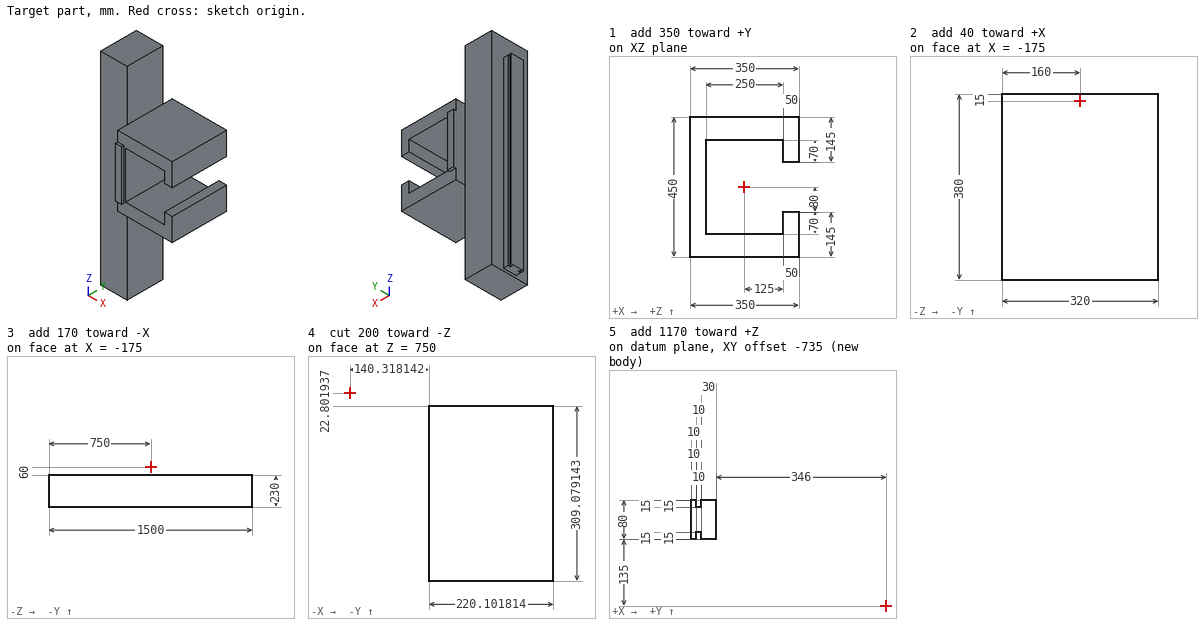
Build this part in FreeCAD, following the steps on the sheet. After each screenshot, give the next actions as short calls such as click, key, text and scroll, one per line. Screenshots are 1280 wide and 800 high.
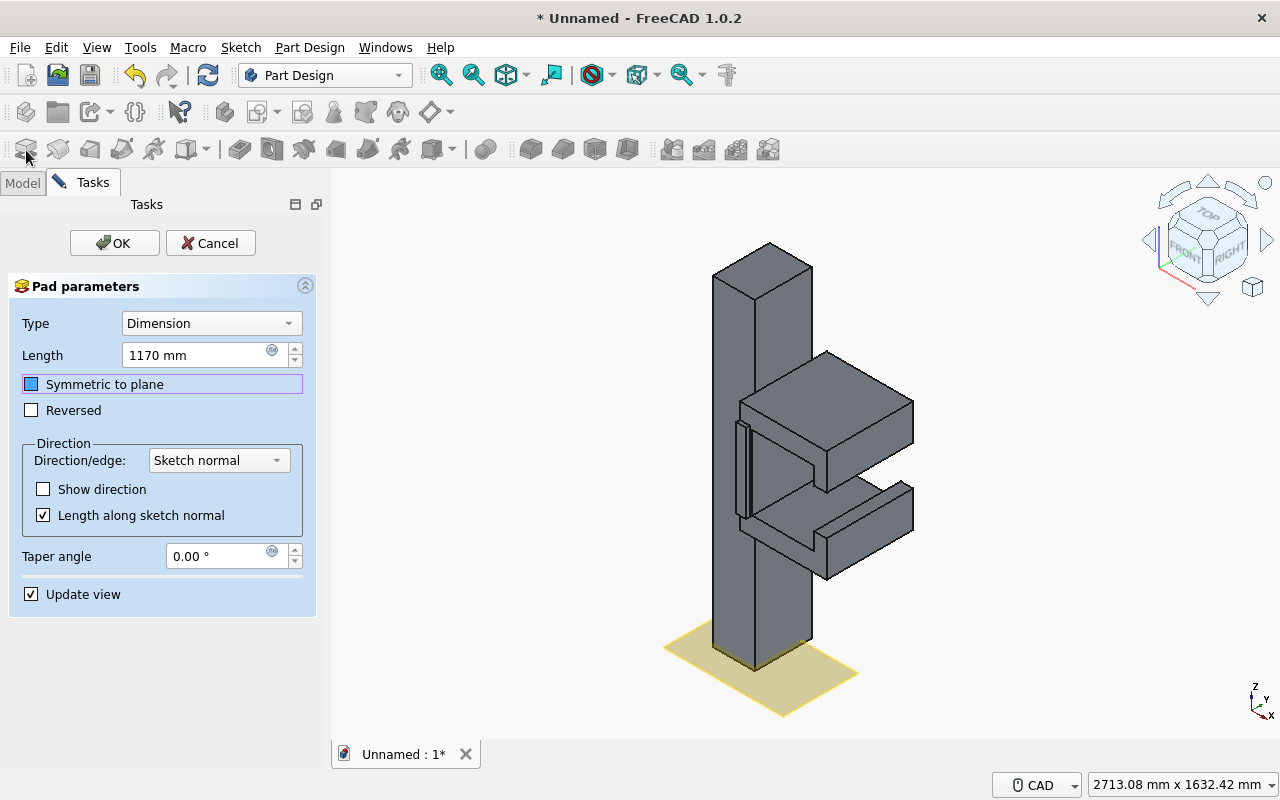
click(115, 243)